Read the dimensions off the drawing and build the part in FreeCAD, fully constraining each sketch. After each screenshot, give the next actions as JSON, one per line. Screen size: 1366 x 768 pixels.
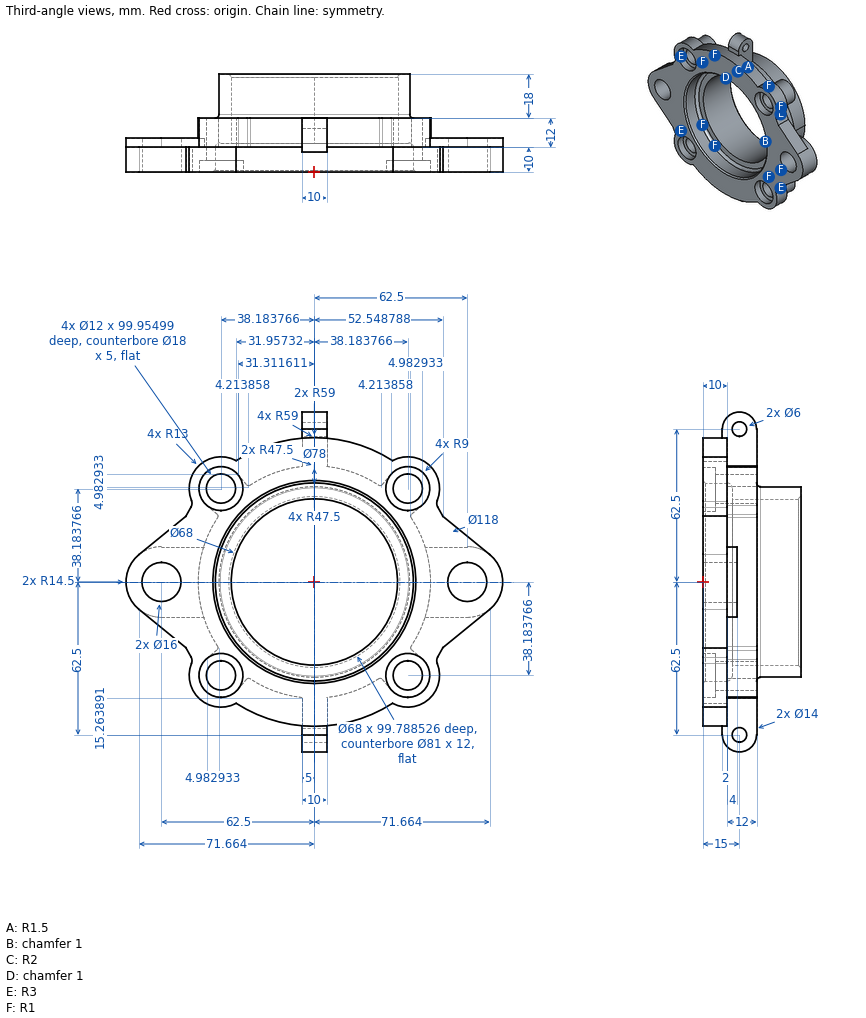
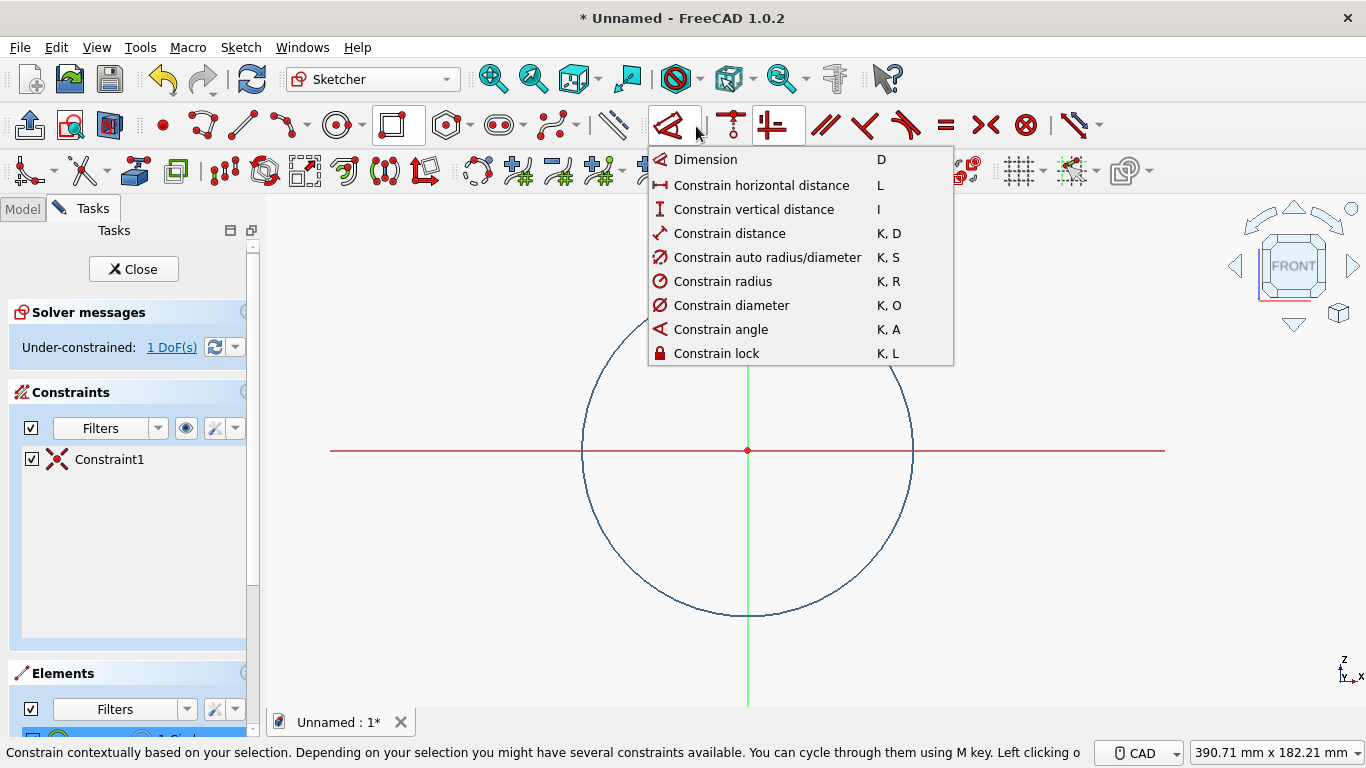
{"action": "left_click", "coordinate": [801, 305]}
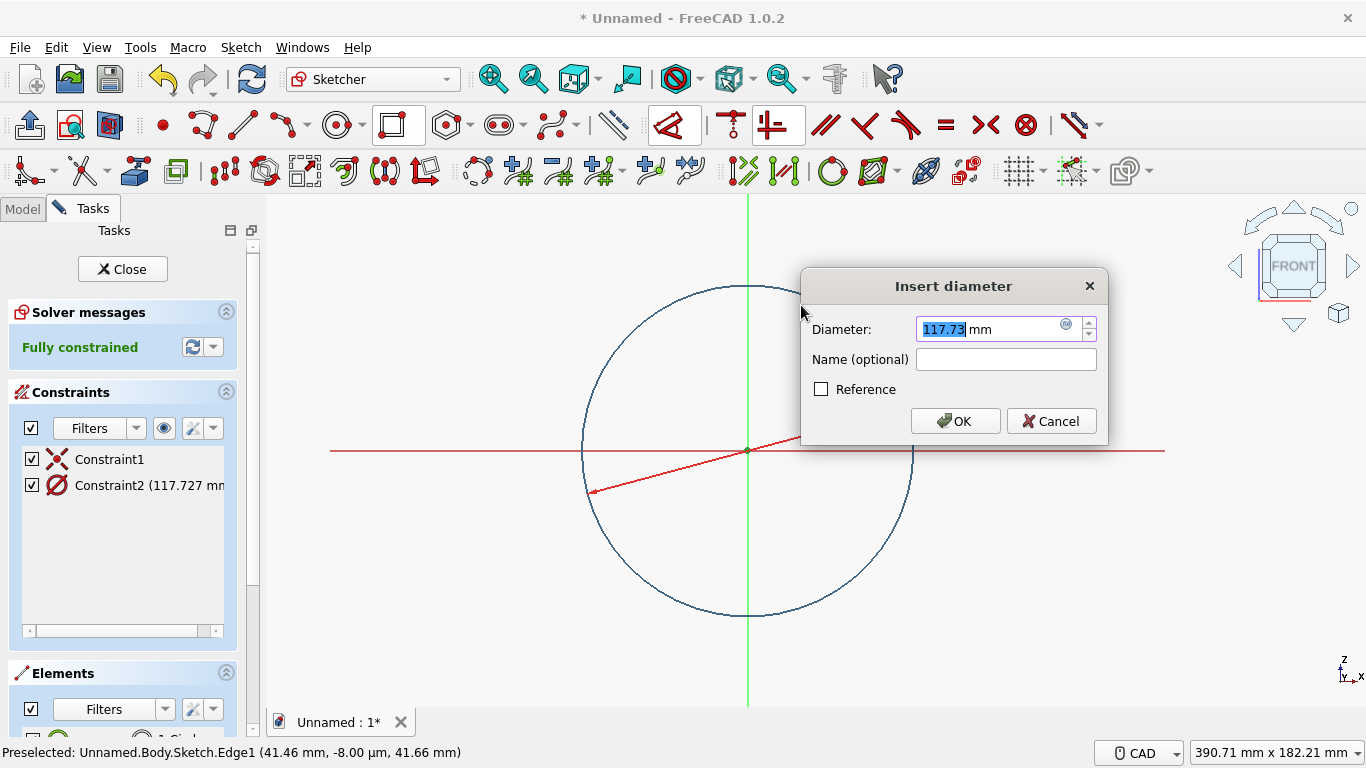
{"action": "type", "text": "118"}
{"action": "key", "text": "Return"}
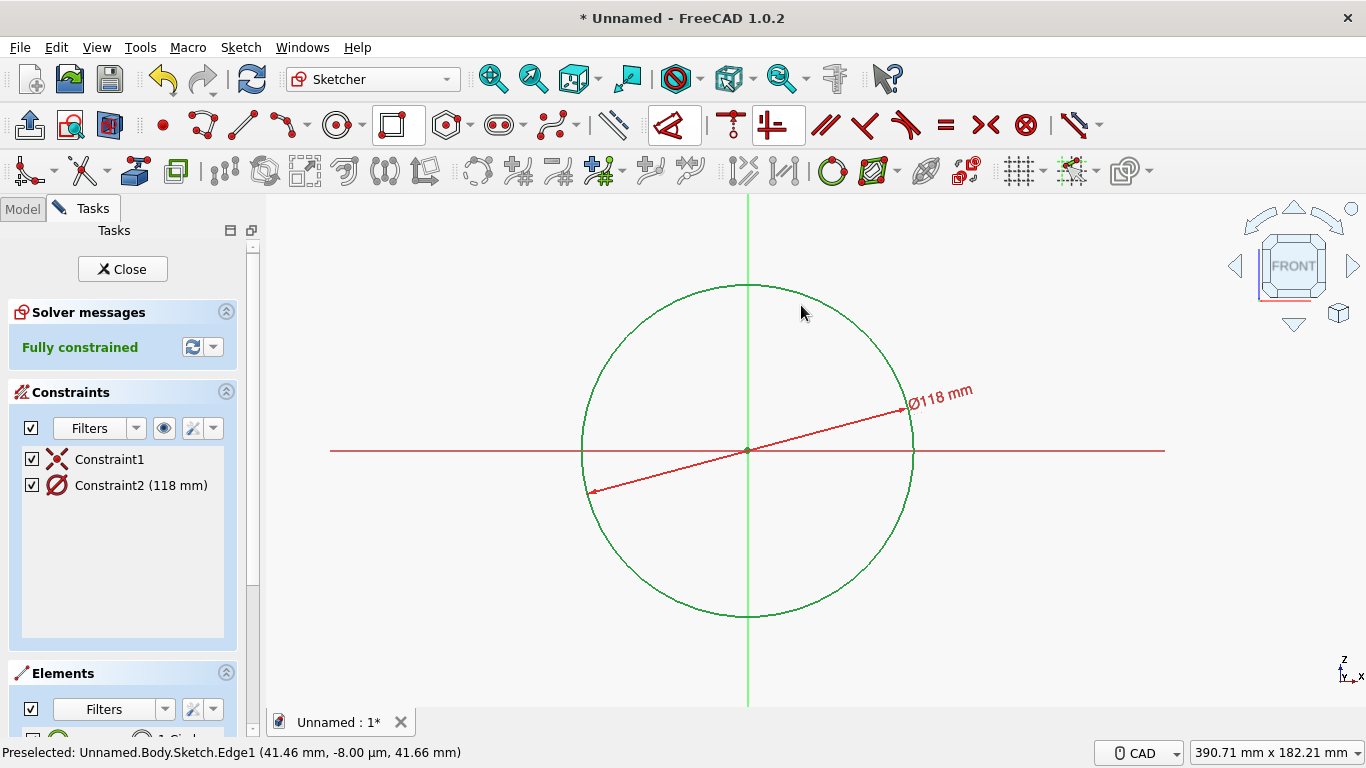
{"action": "left_click", "coordinate": [123, 269]}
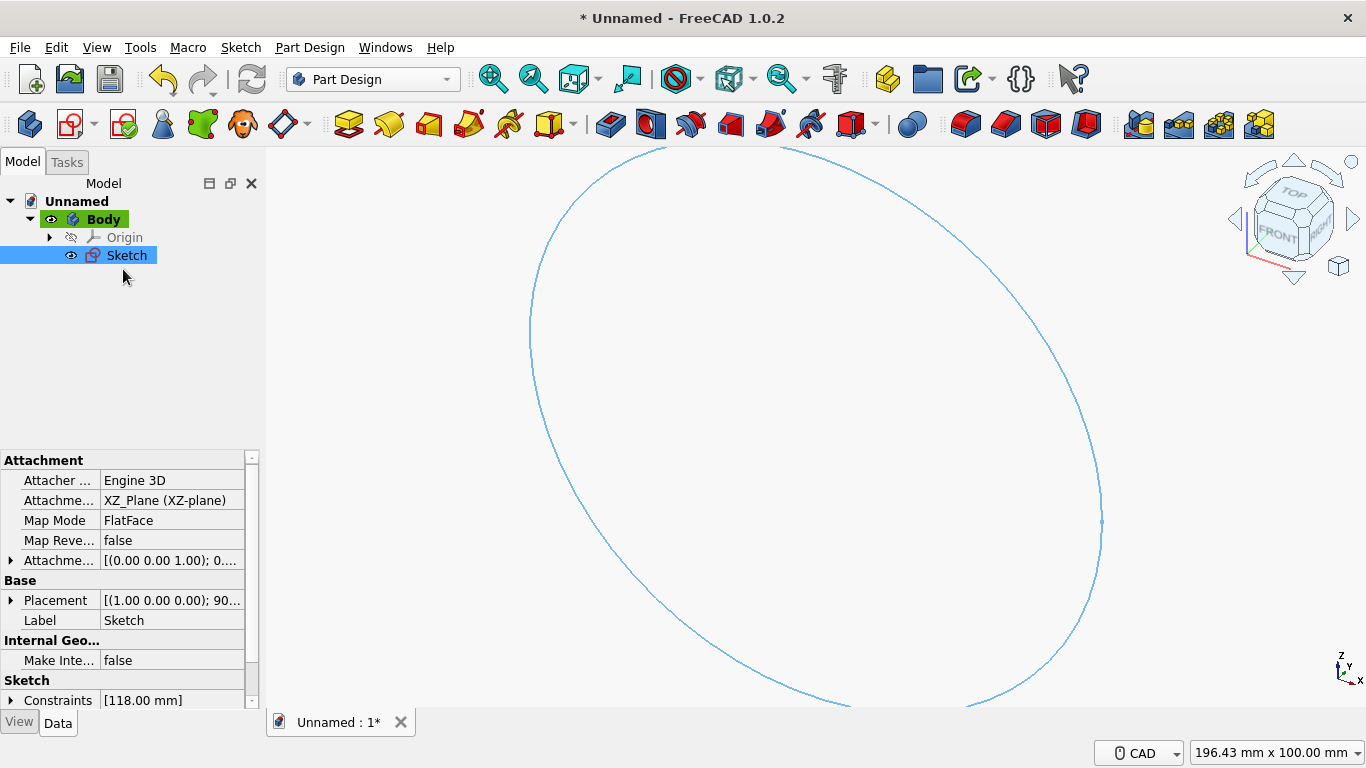
{"action": "left_click", "coordinate": [350, 124]}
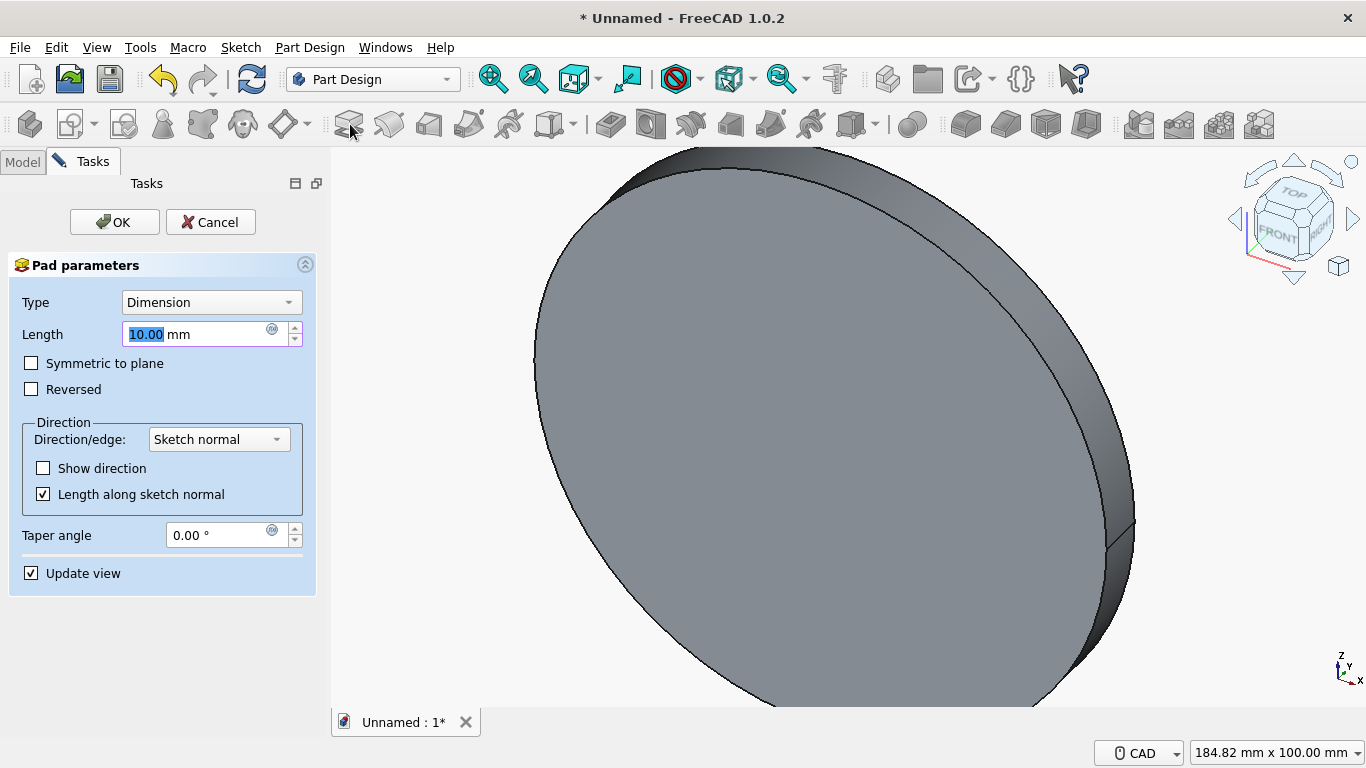
{"action": "type", "text": "10"}
{"action": "key", "text": "Tab"}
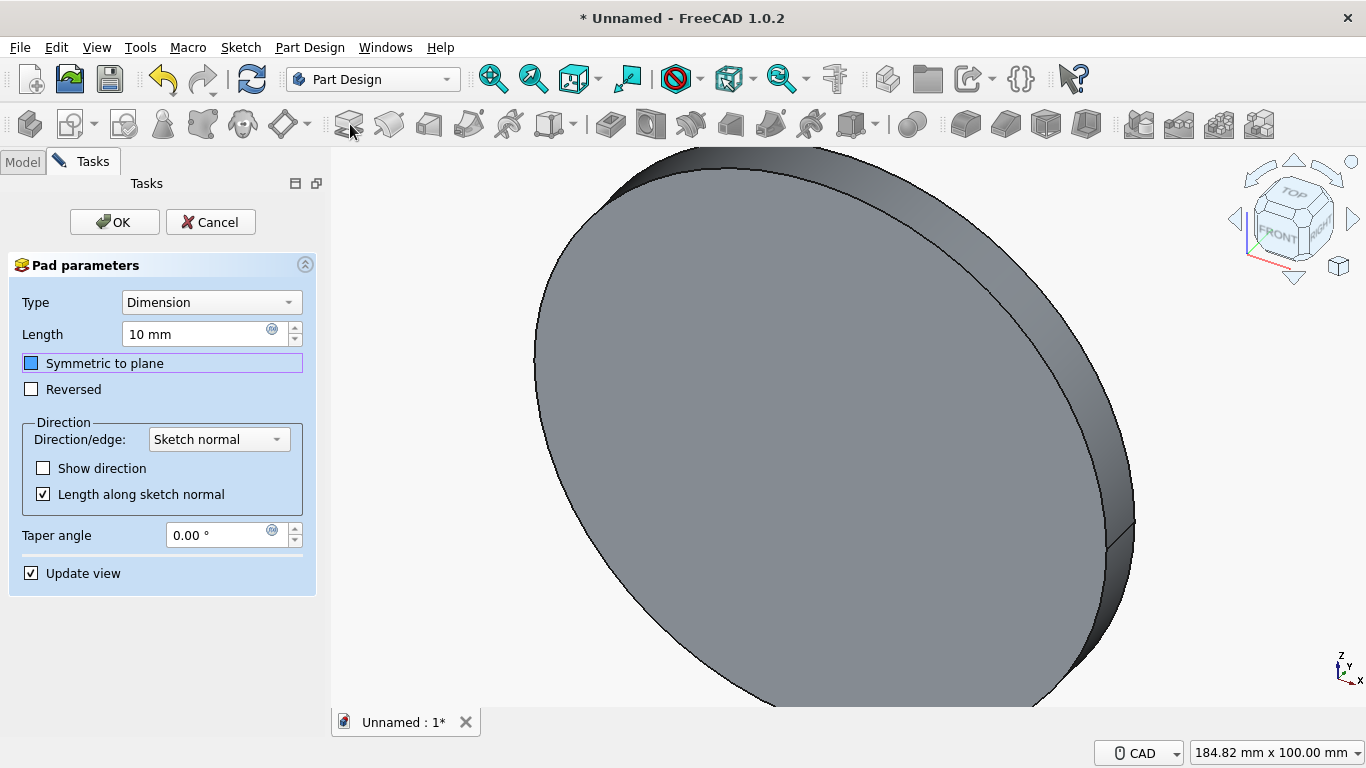
{"action": "left_click", "coordinate": [30, 389]}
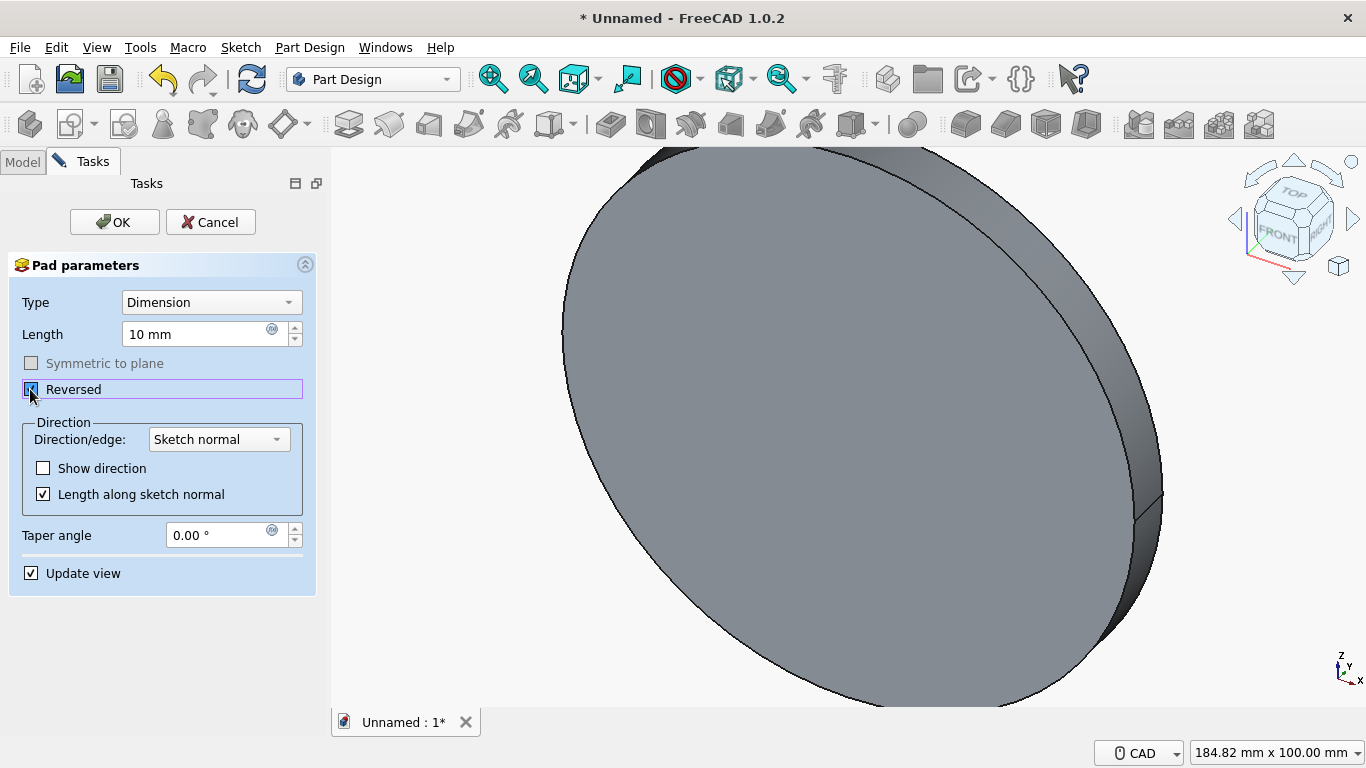
{"action": "left_click", "coordinate": [115, 222]}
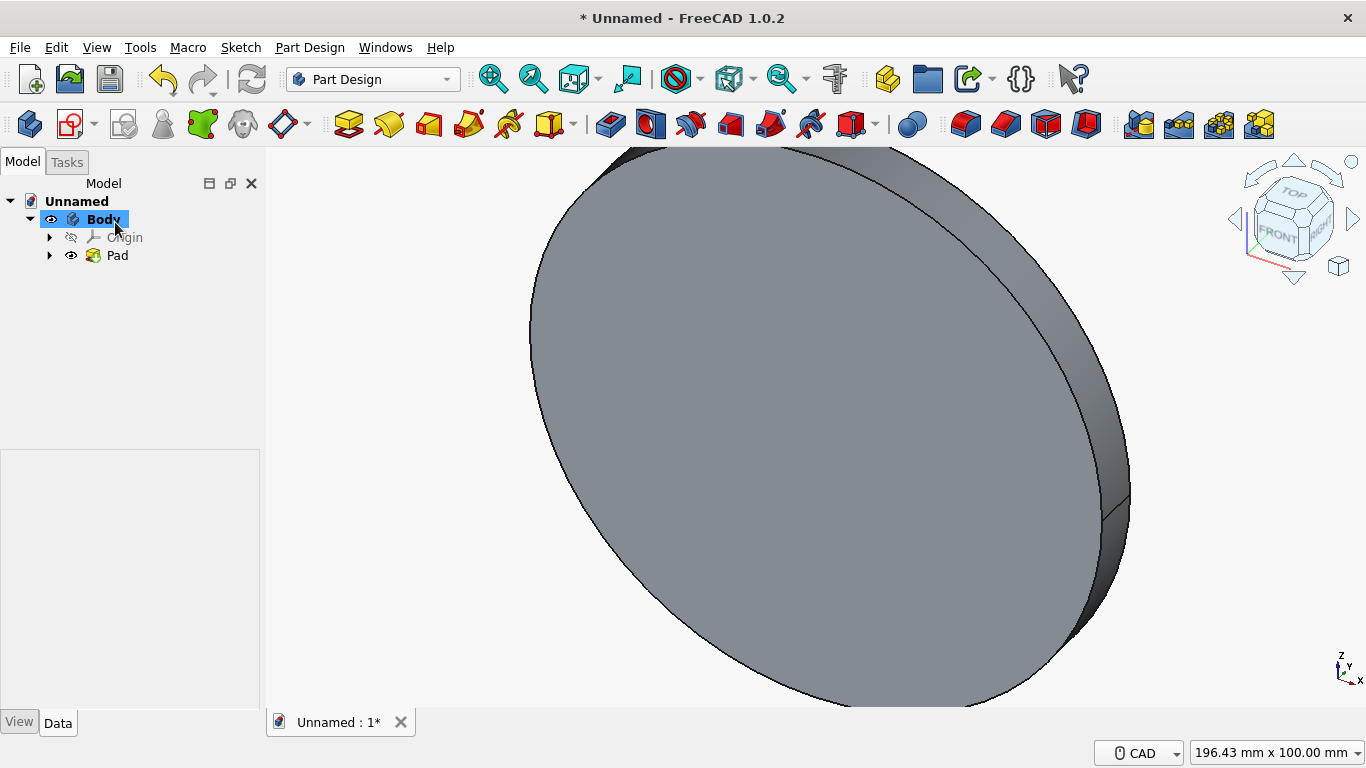
{"action": "left_click", "coordinate": [494, 80]}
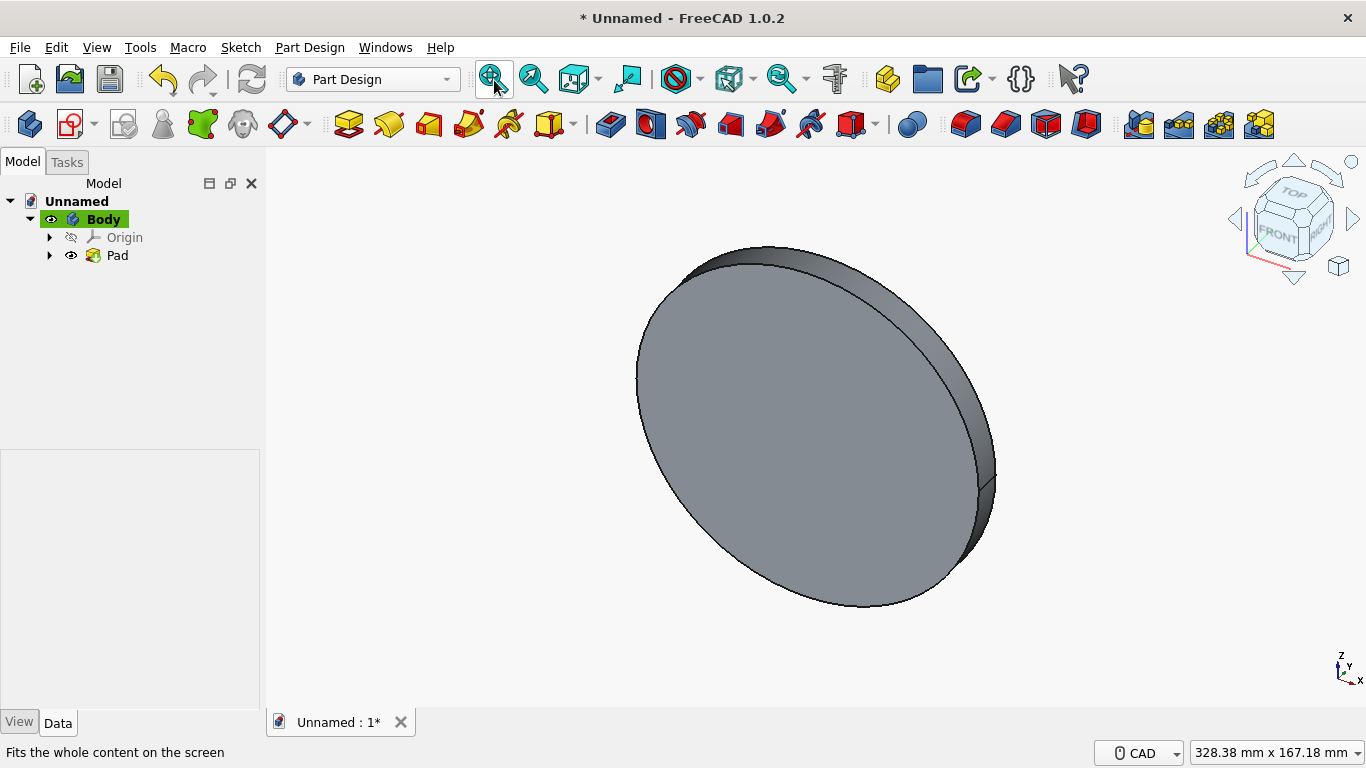
{"action": "left_click", "coordinate": [808, 434]}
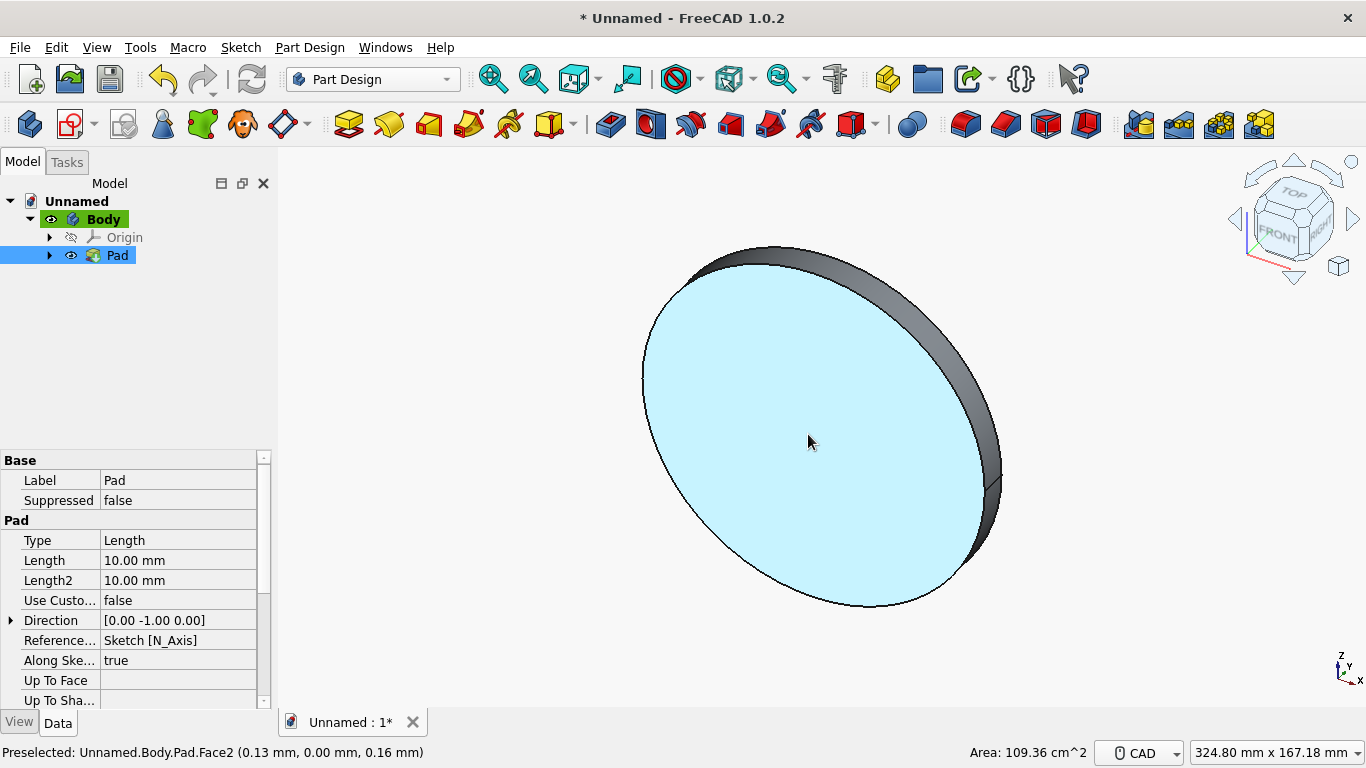
{"action": "left_click", "coordinate": [70, 124]}